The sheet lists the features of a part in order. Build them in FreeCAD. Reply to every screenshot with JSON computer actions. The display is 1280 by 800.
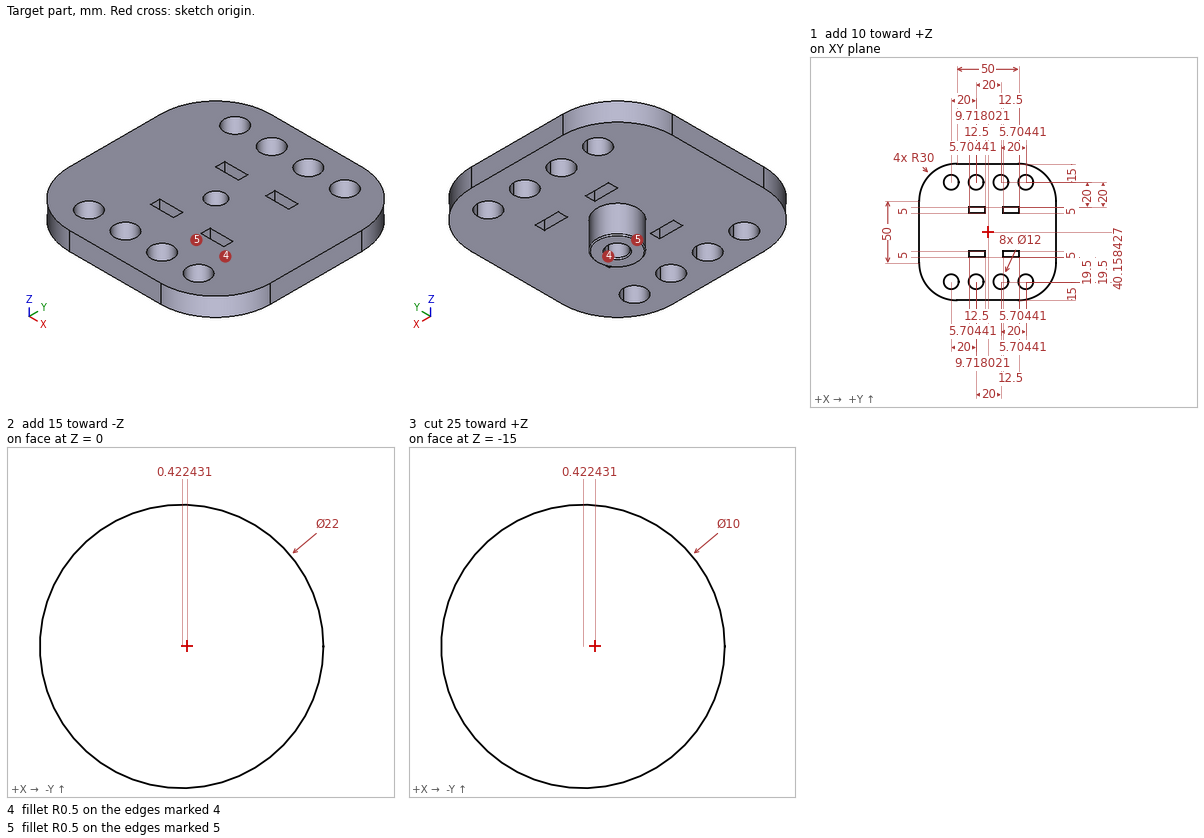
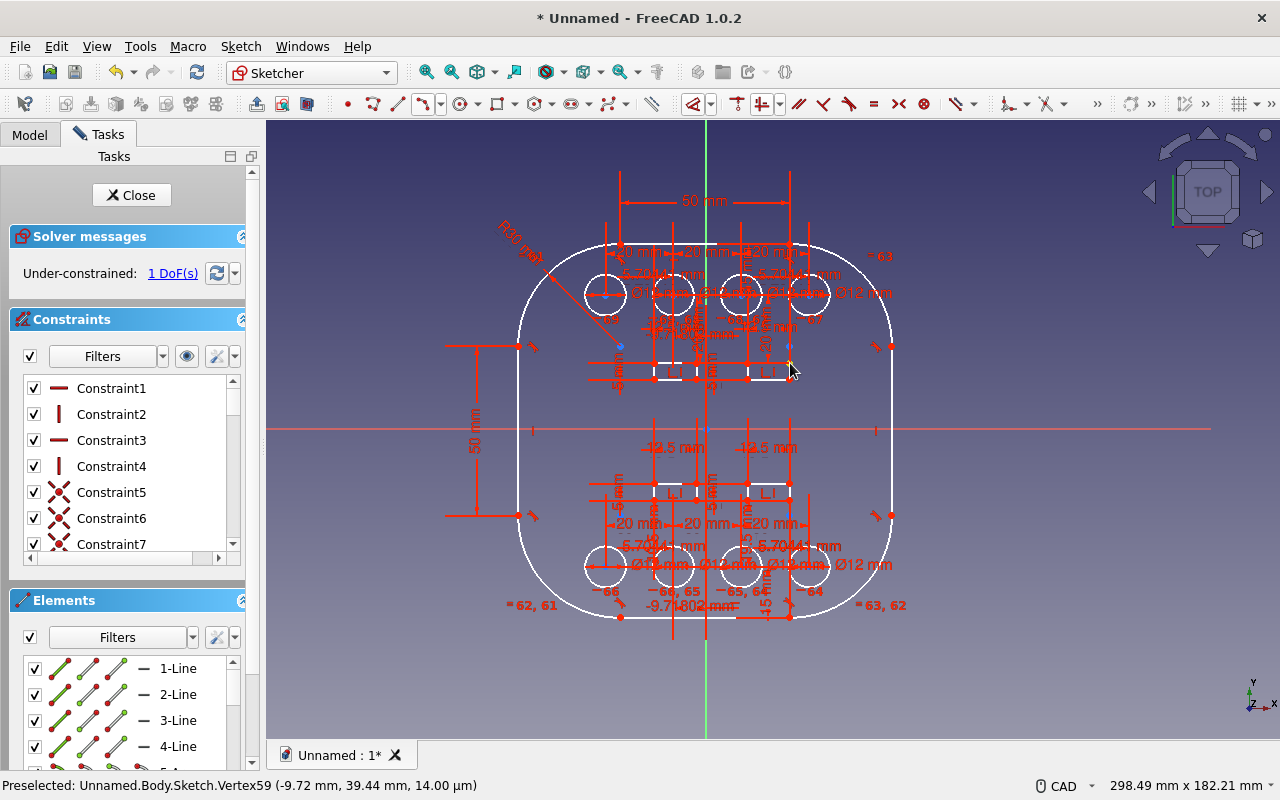
{"action": "left_click", "coordinate": [809, 567]}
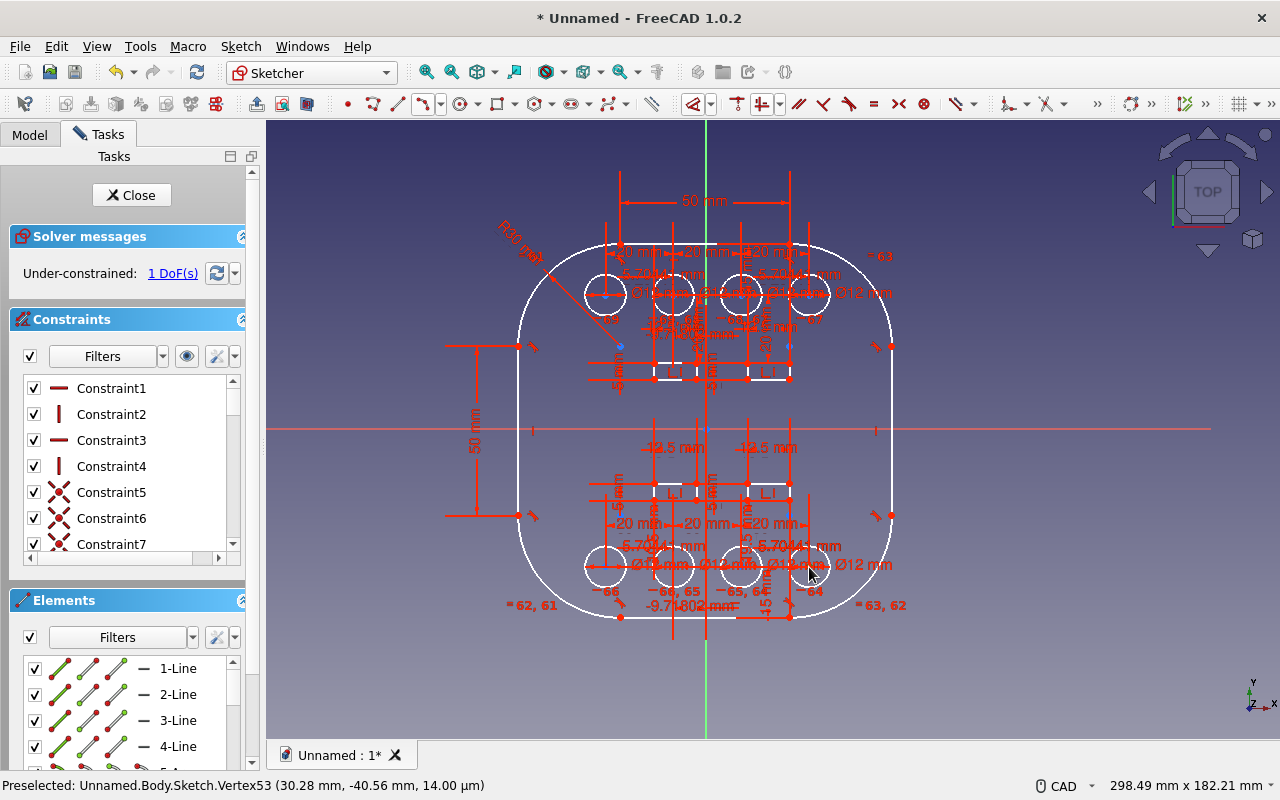
{"action": "key", "text": "i"}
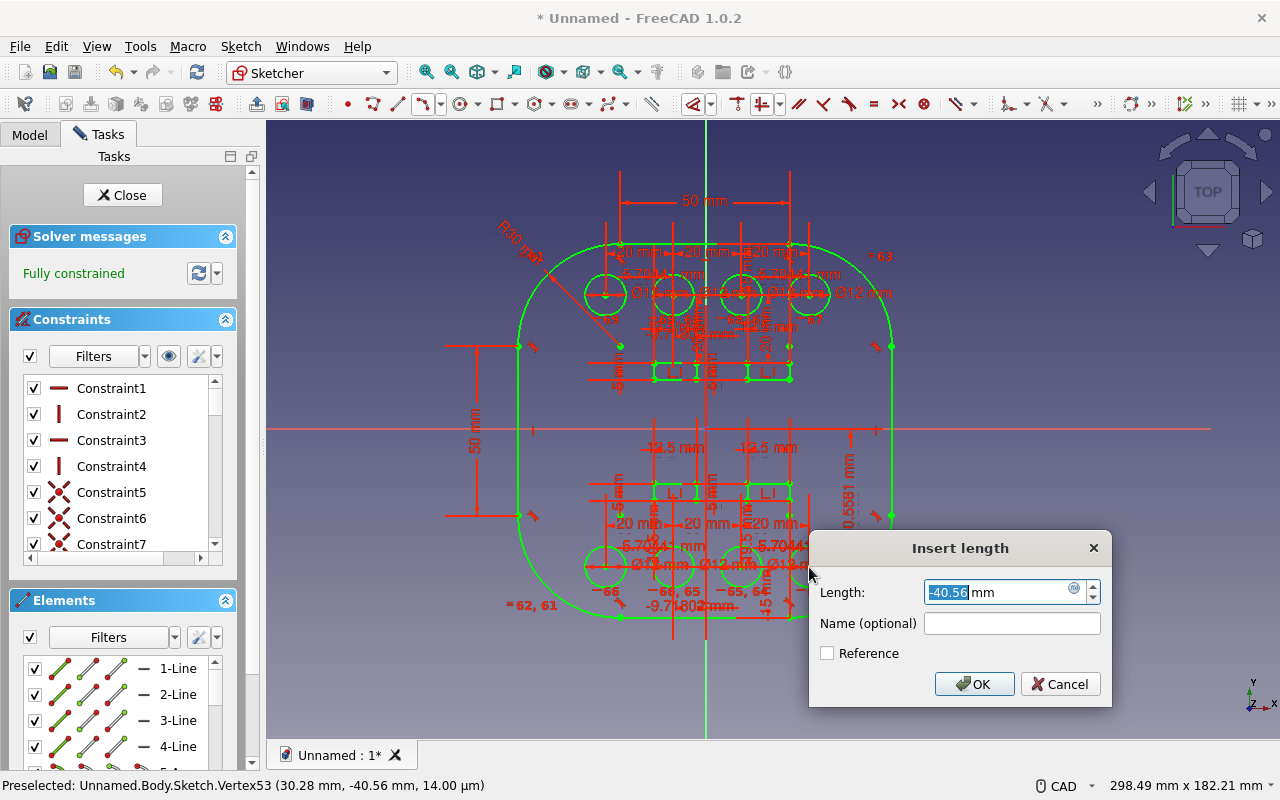
{"action": "type", "text": "-40.158427"}
{"action": "key", "text": "Return"}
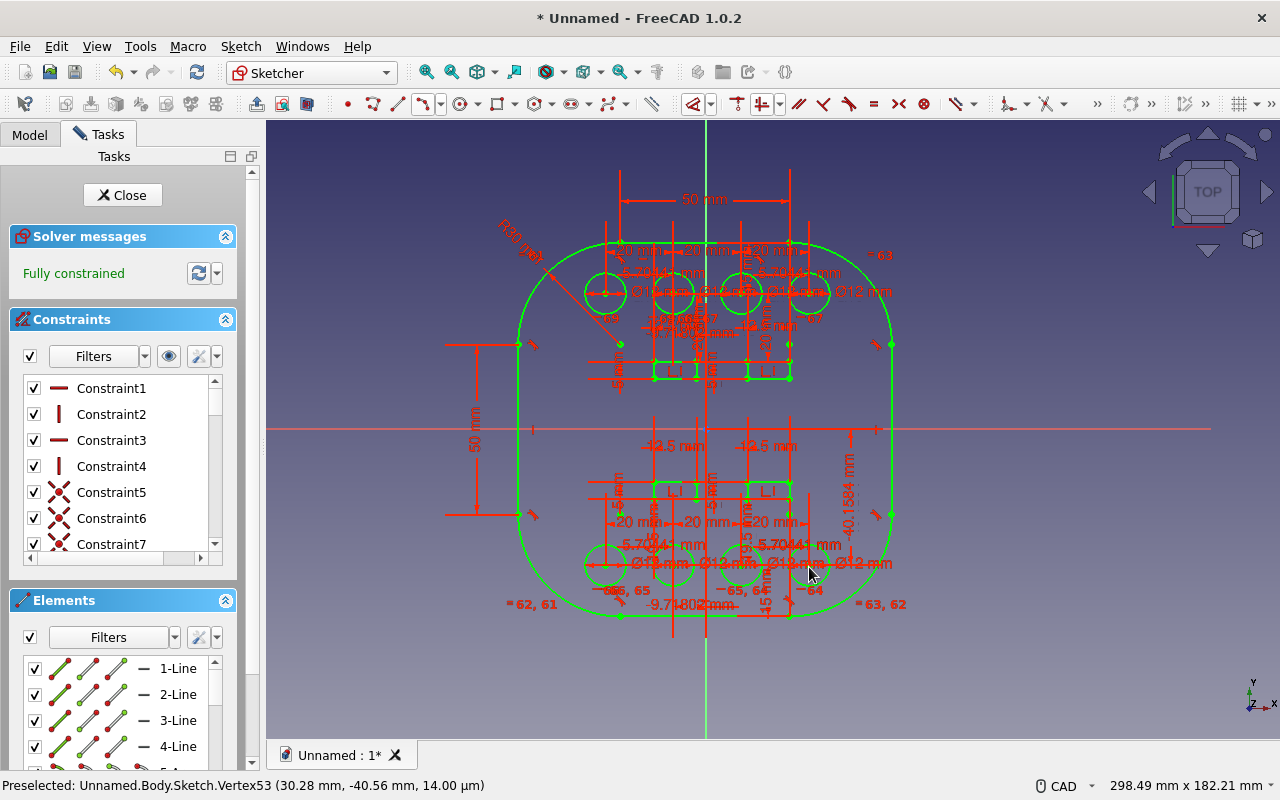
{"action": "left_click", "coordinate": [123, 195]}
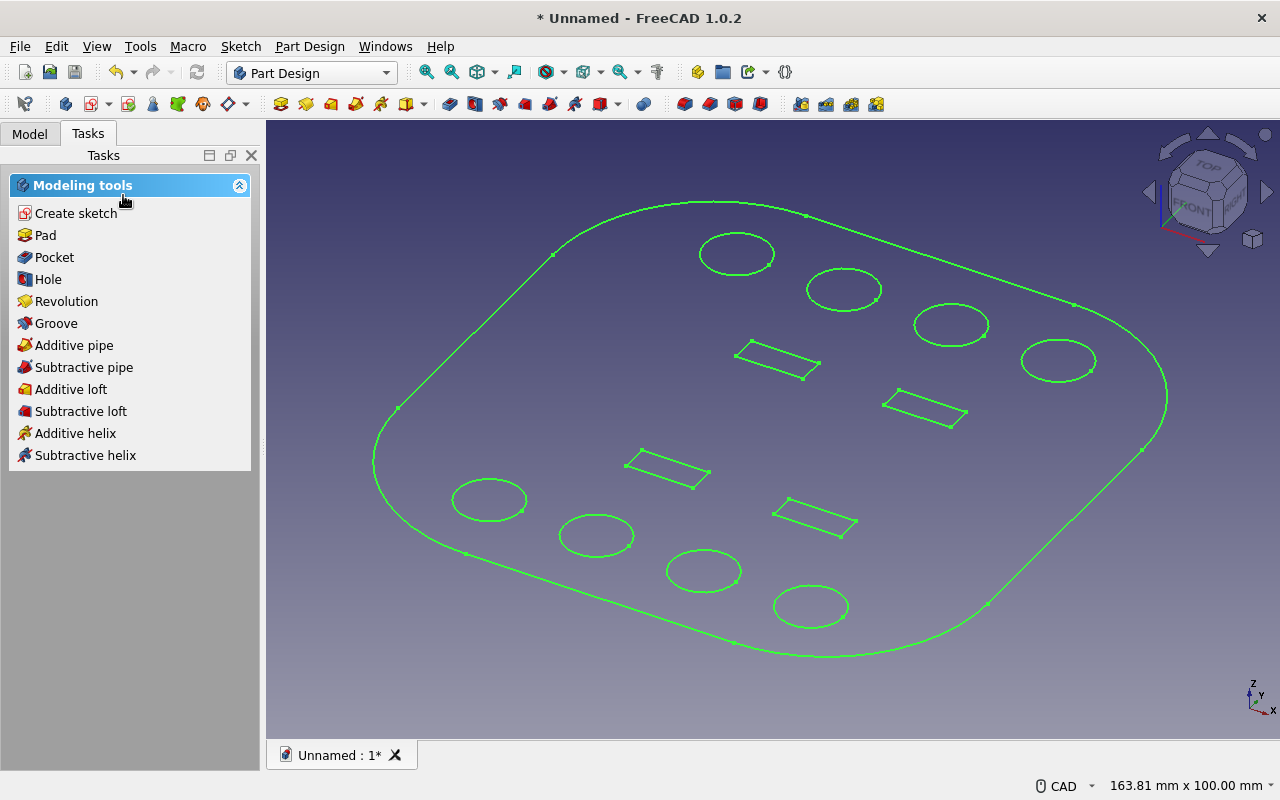
{"action": "left_click", "coordinate": [281, 104]}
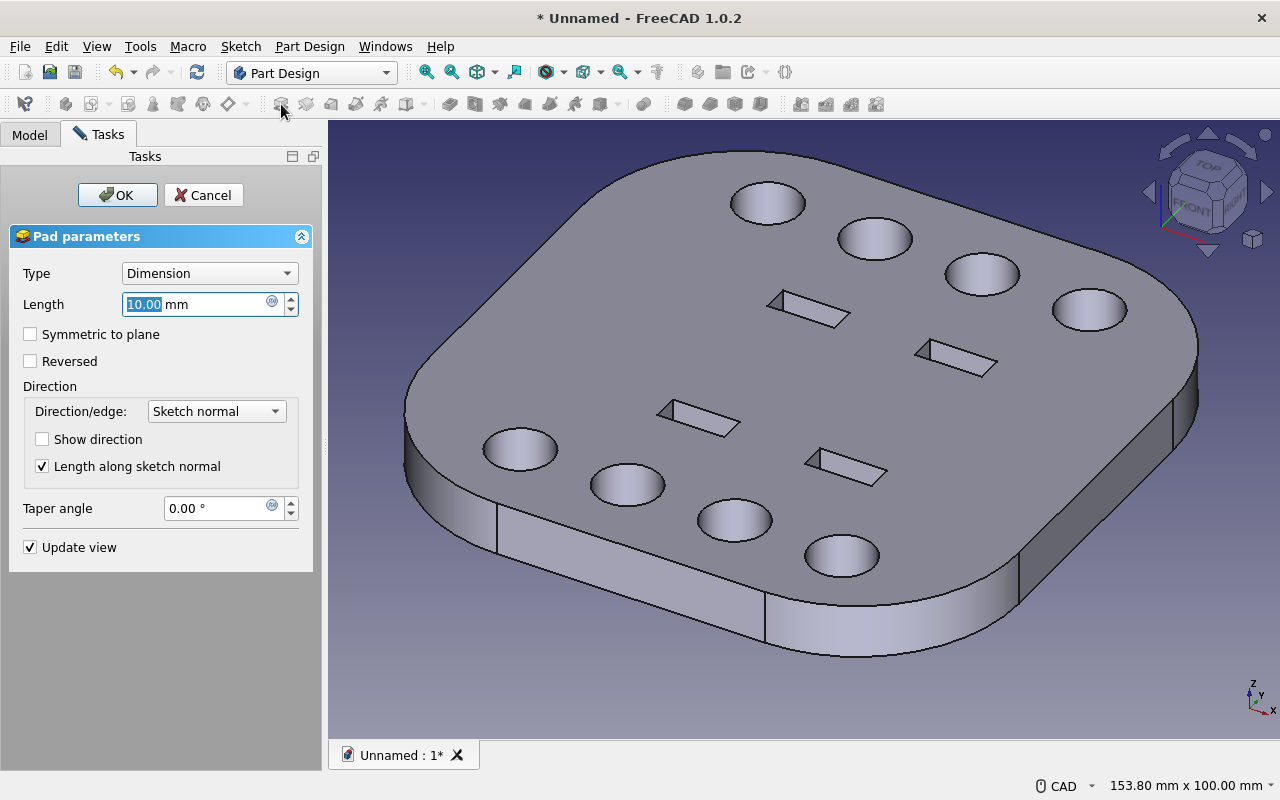
{"action": "type", "text": "10"}
{"action": "key", "text": "Tab"}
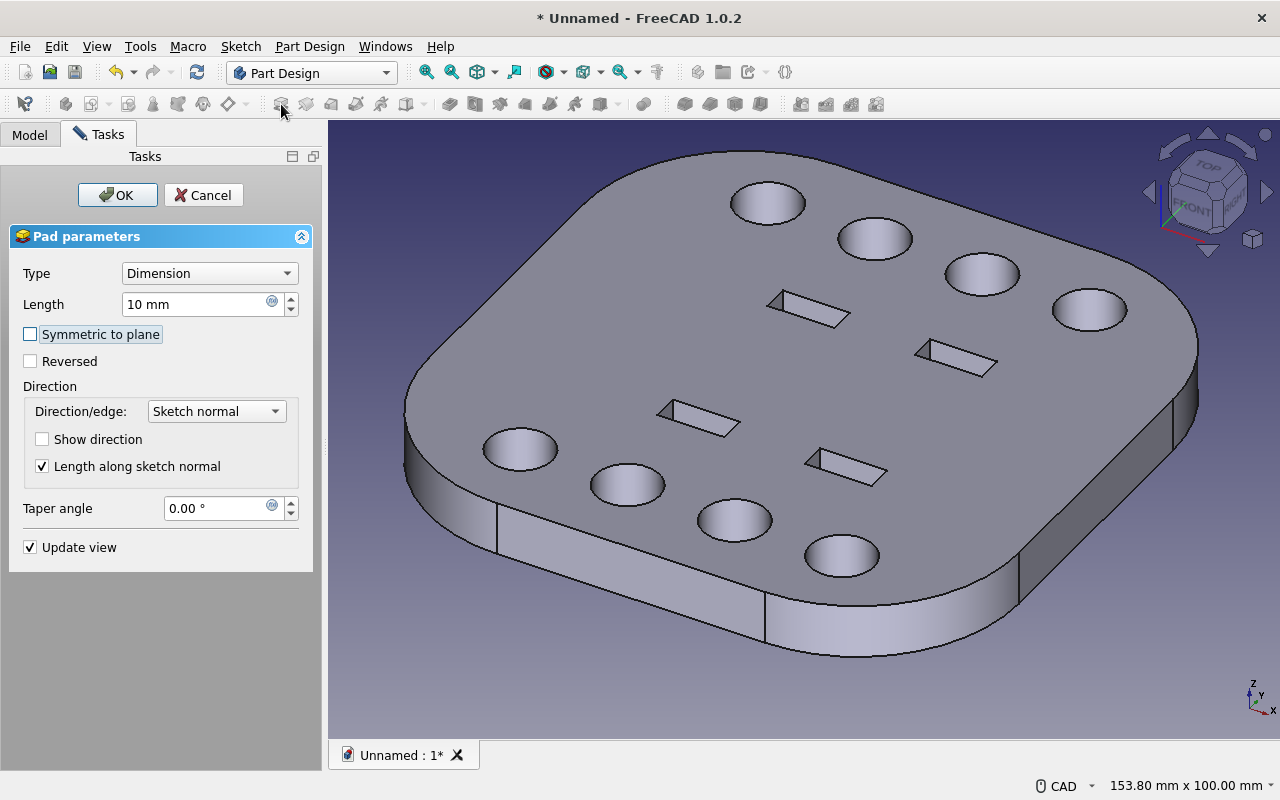
{"action": "left_click", "coordinate": [118, 195]}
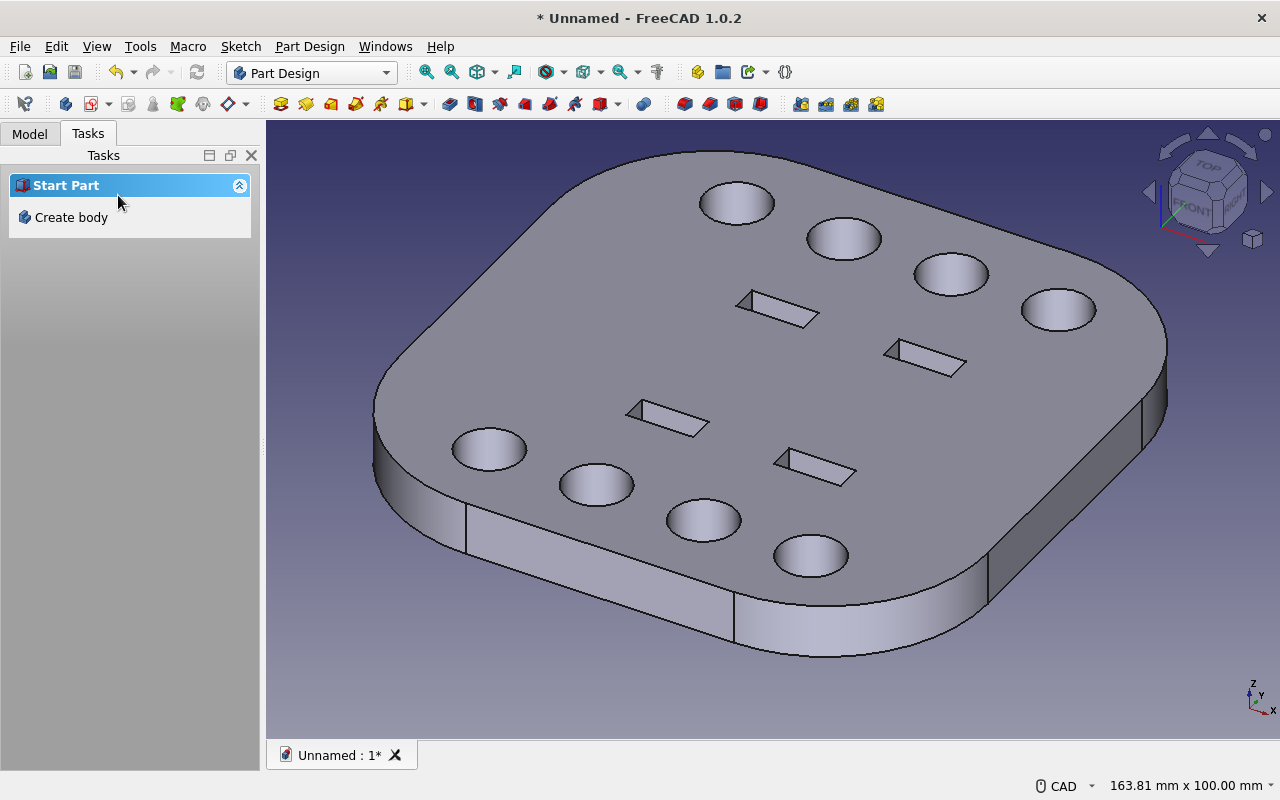
{"action": "left_click", "coordinate": [427, 72]}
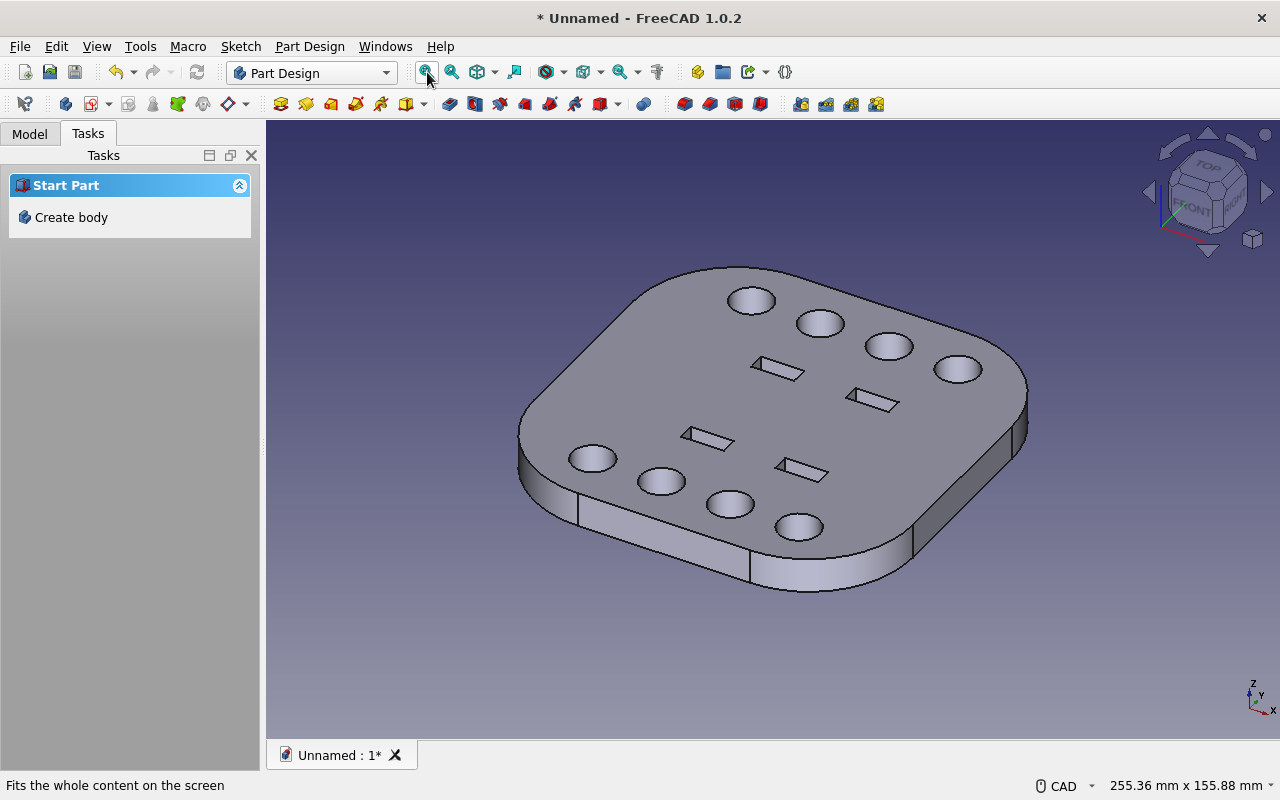
{"action": "key", "text": "5"}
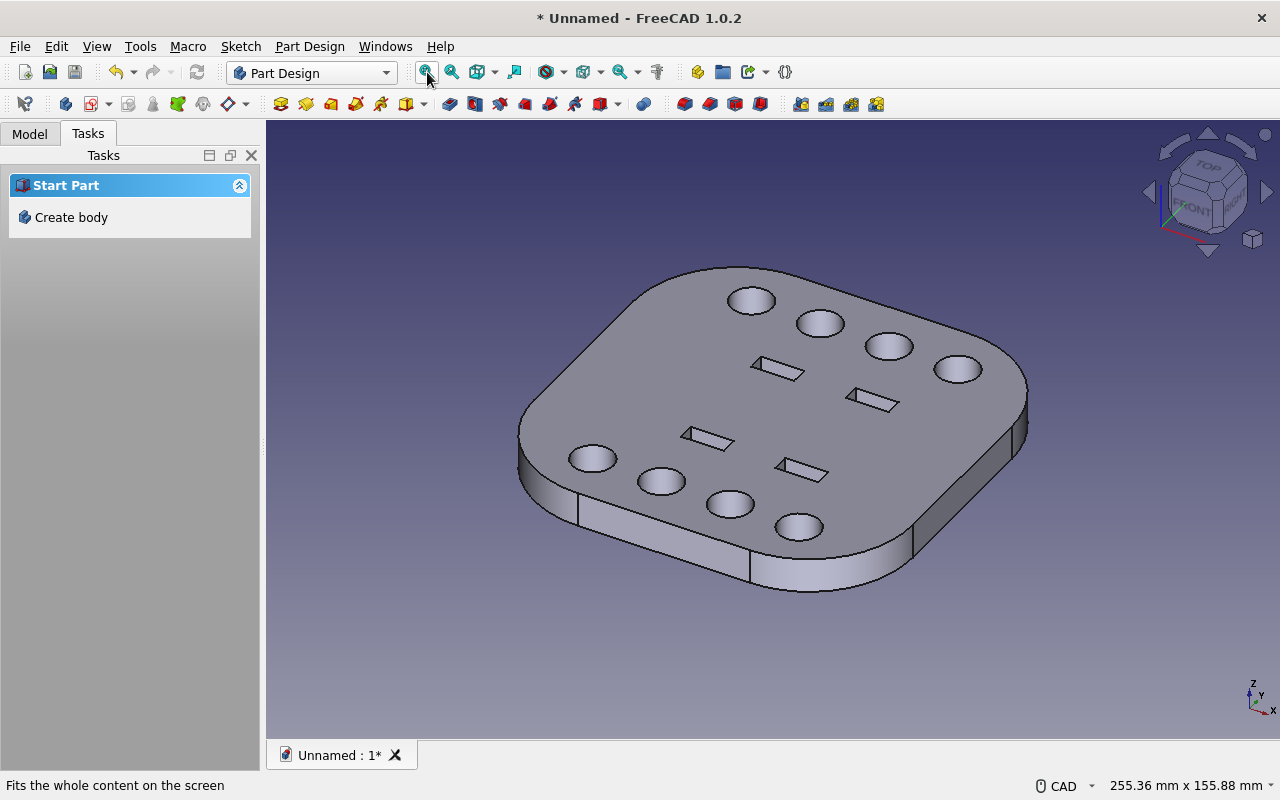
{"action": "left_click", "coordinate": [648, 428]}